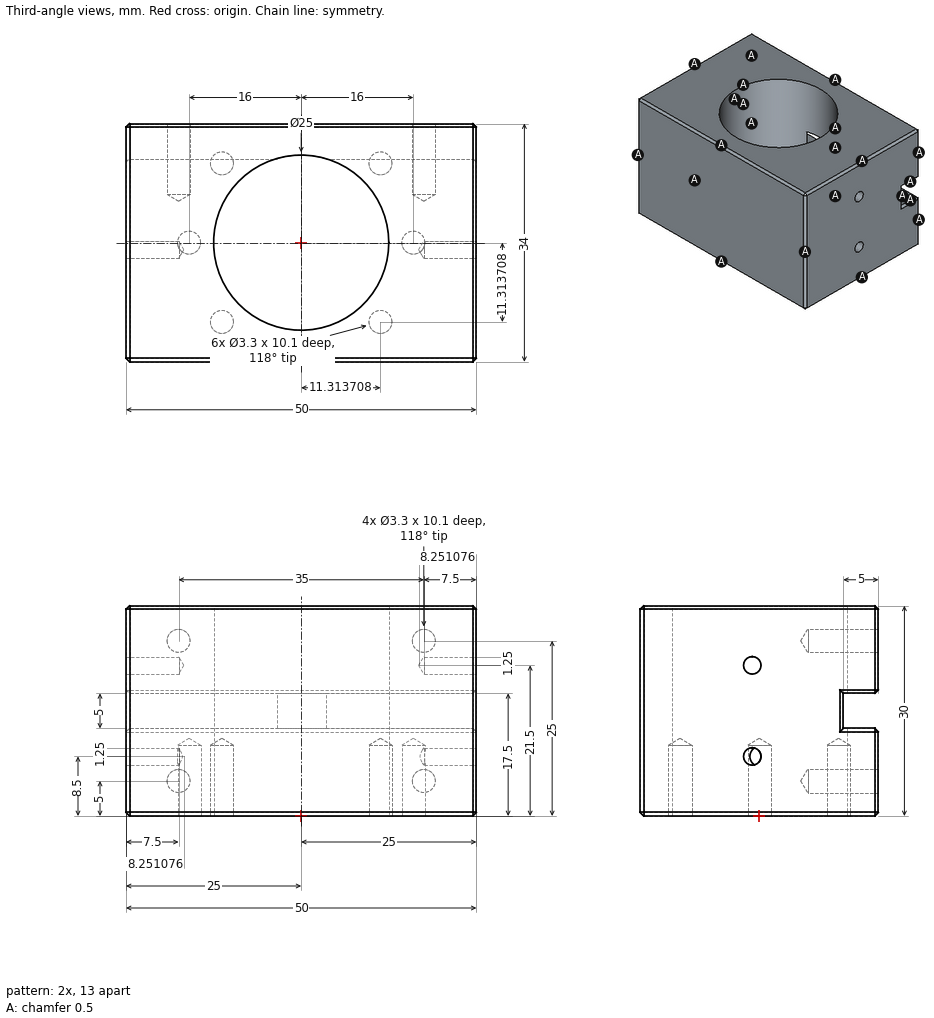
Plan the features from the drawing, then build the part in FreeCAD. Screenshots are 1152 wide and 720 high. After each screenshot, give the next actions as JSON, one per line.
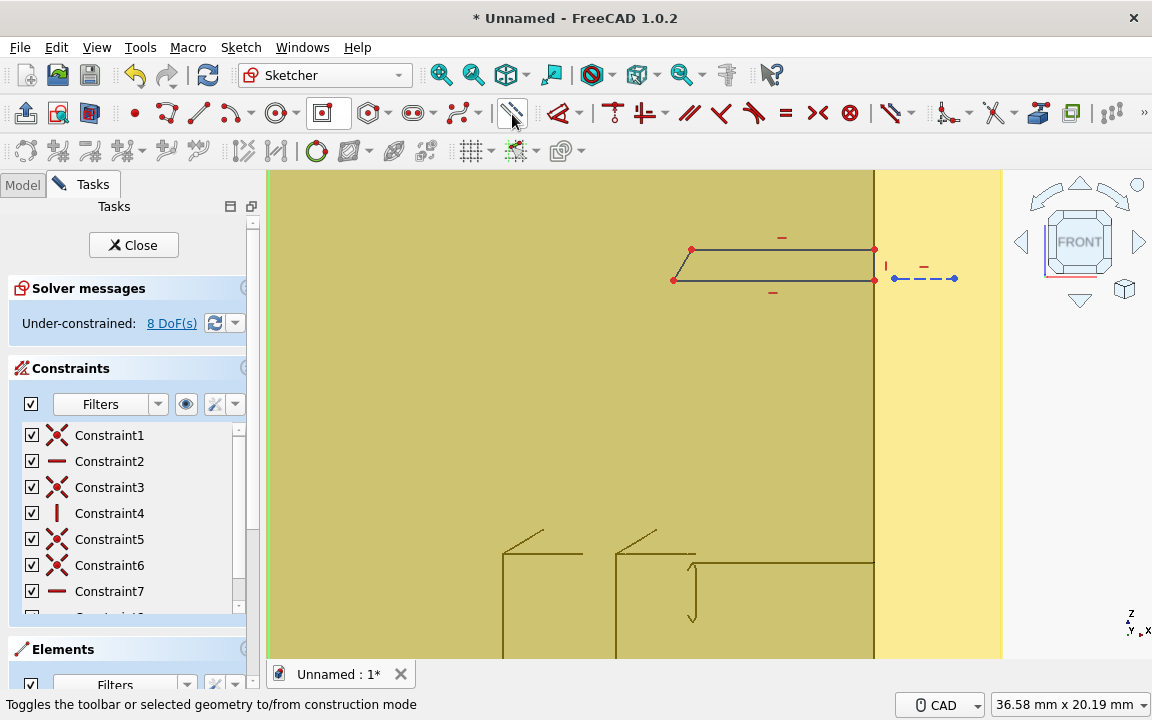
{"action": "left_click", "coordinate": [747, 250]}
{"action": "left_click", "coordinate": [783, 216]}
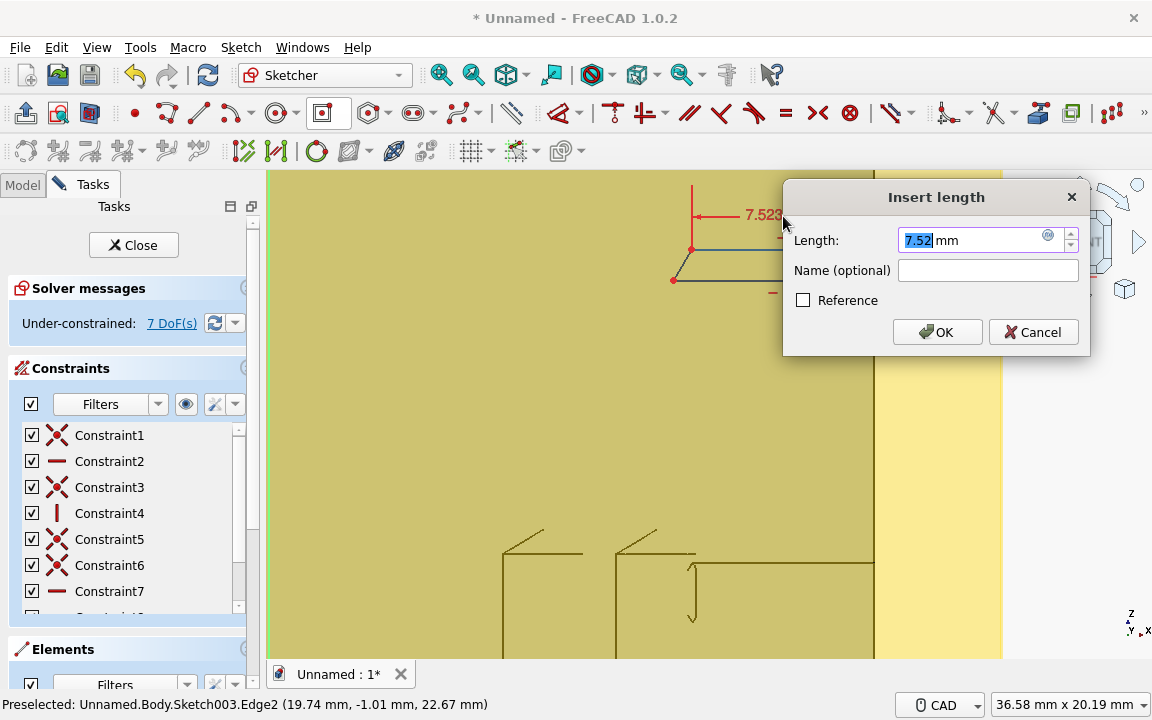
{"action": "type", "text": "7.5"}
{"action": "key", "text": "Return"}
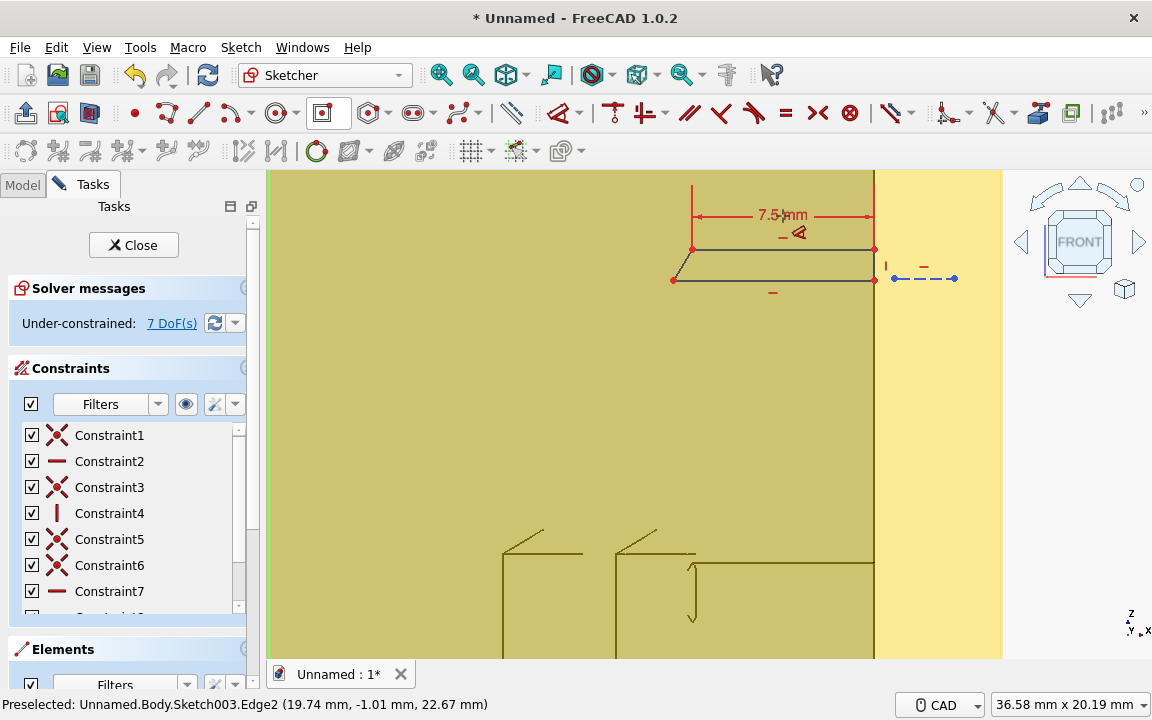
{"action": "left_click", "coordinate": [874, 250]}
{"action": "left_click", "coordinate": [584, 216]}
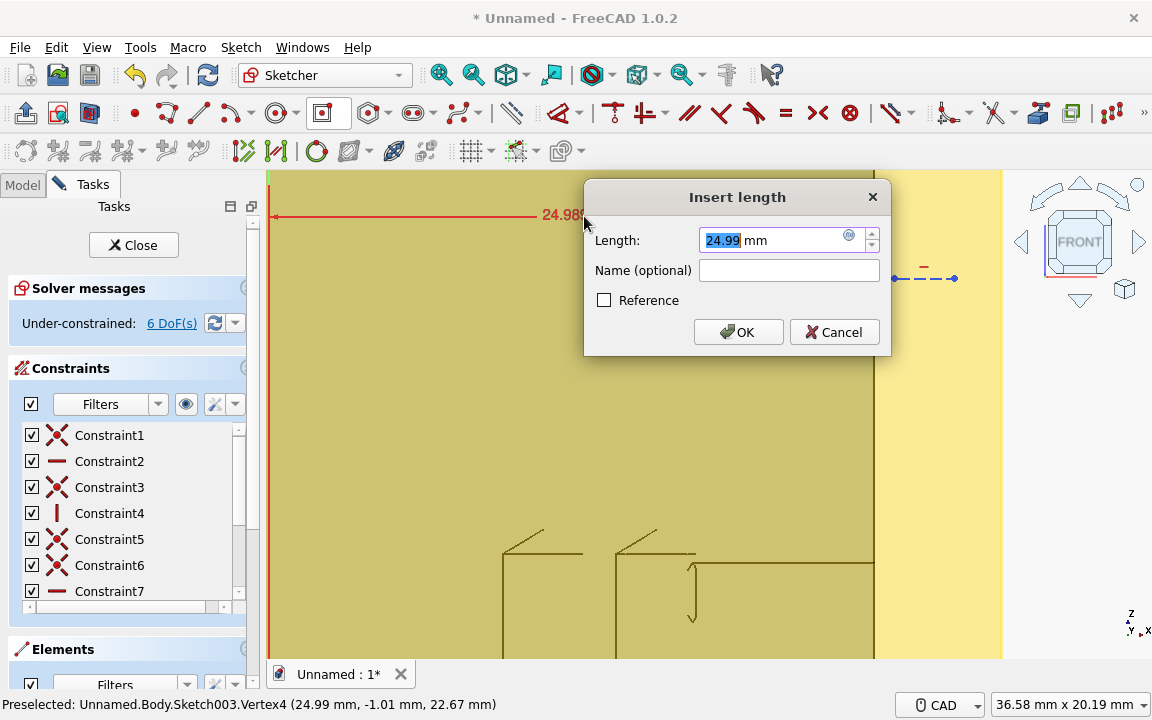
{"action": "type", "text": "25"}
{"action": "key", "text": "Return"}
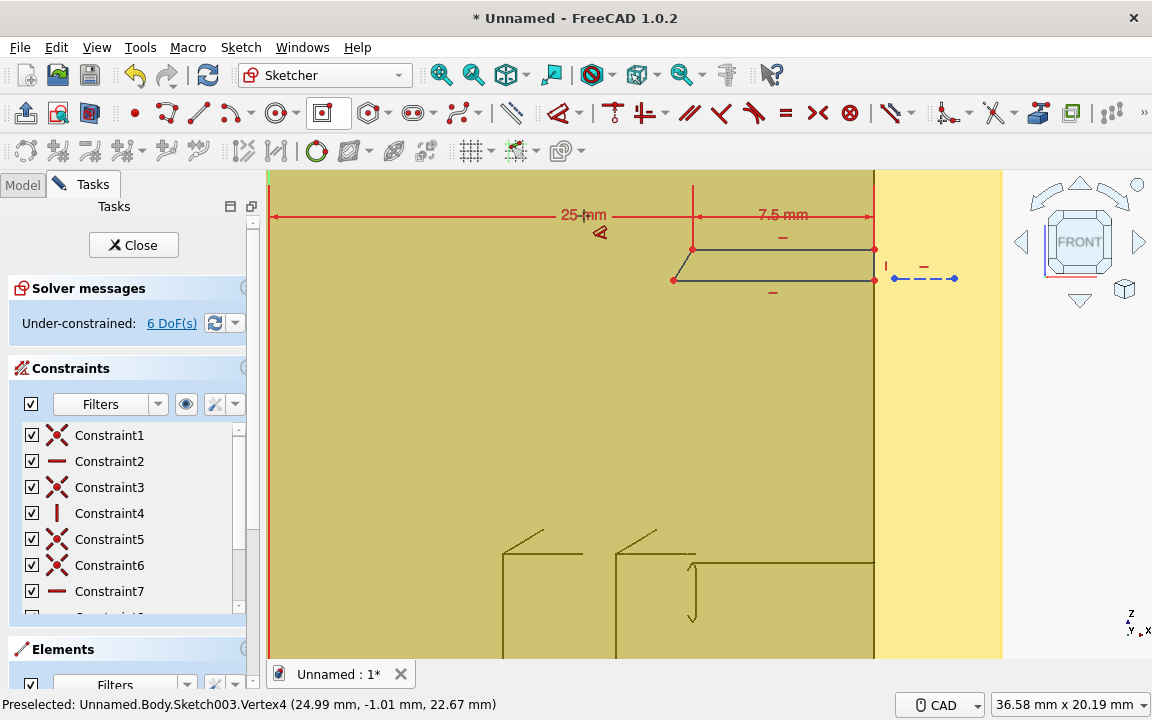
{"action": "scroll", "coordinate": [874, 259], "scroll_direction": "up", "scroll_amount": 2}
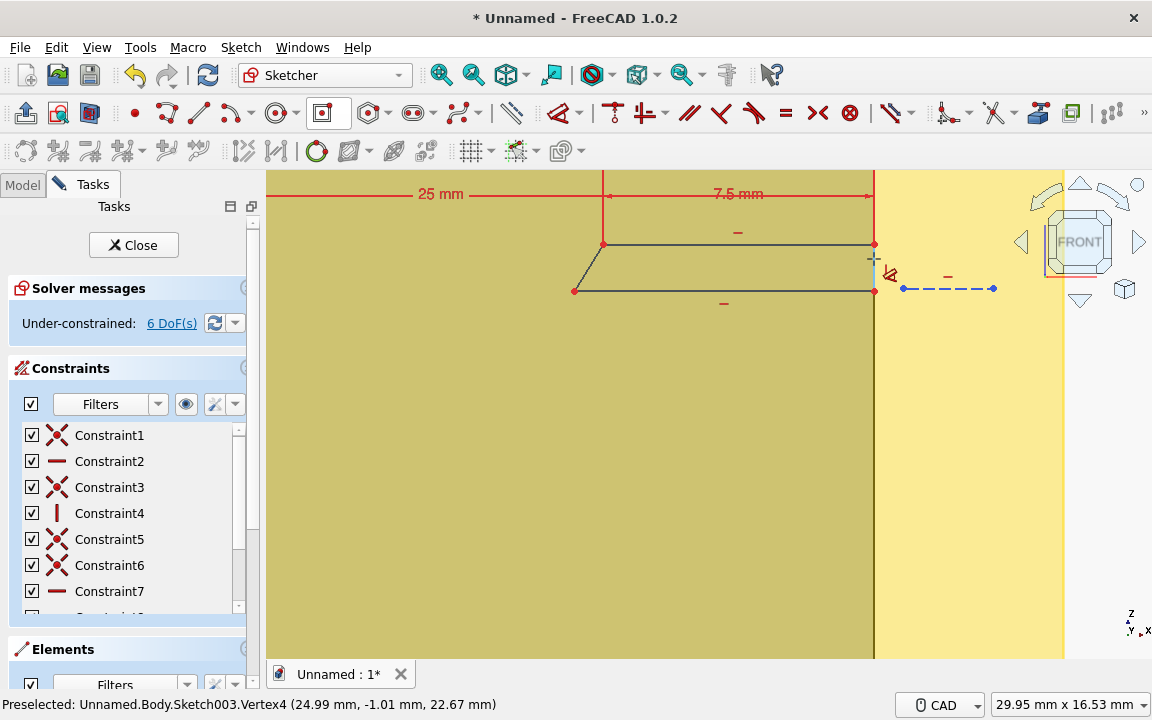
{"action": "left_click", "coordinate": [874, 259]}
{"action": "left_click", "coordinate": [908, 268]}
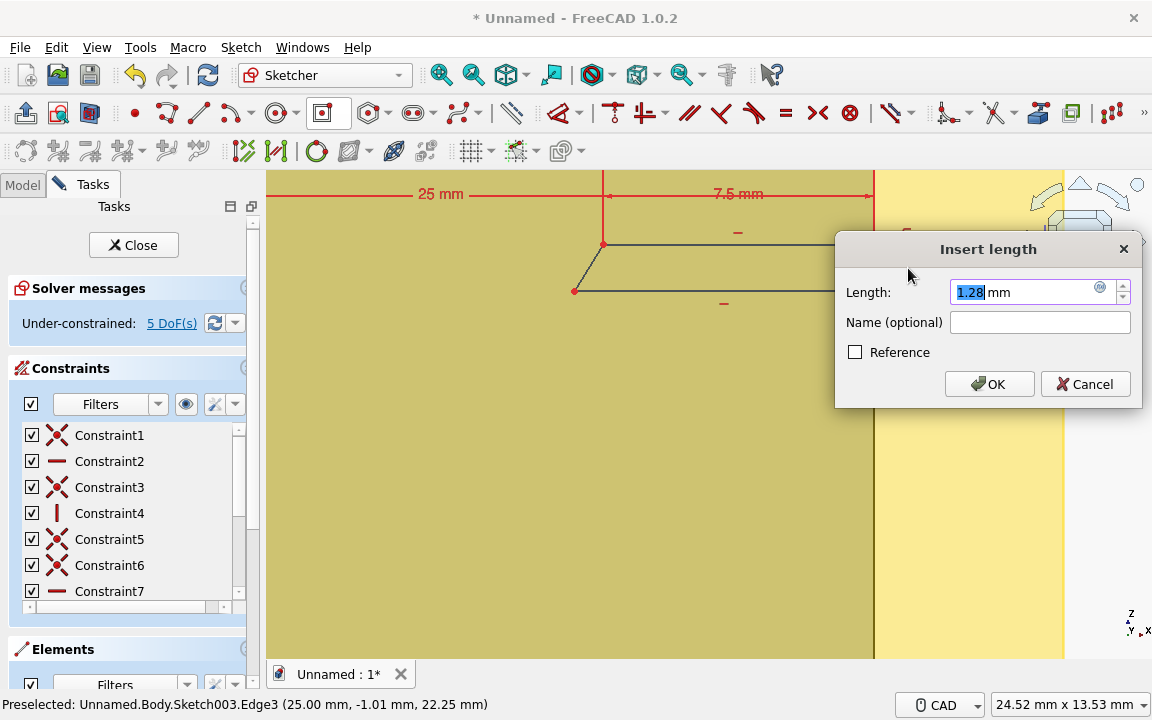
{"action": "type", "text": "1.25"}
{"action": "key", "text": "Return"}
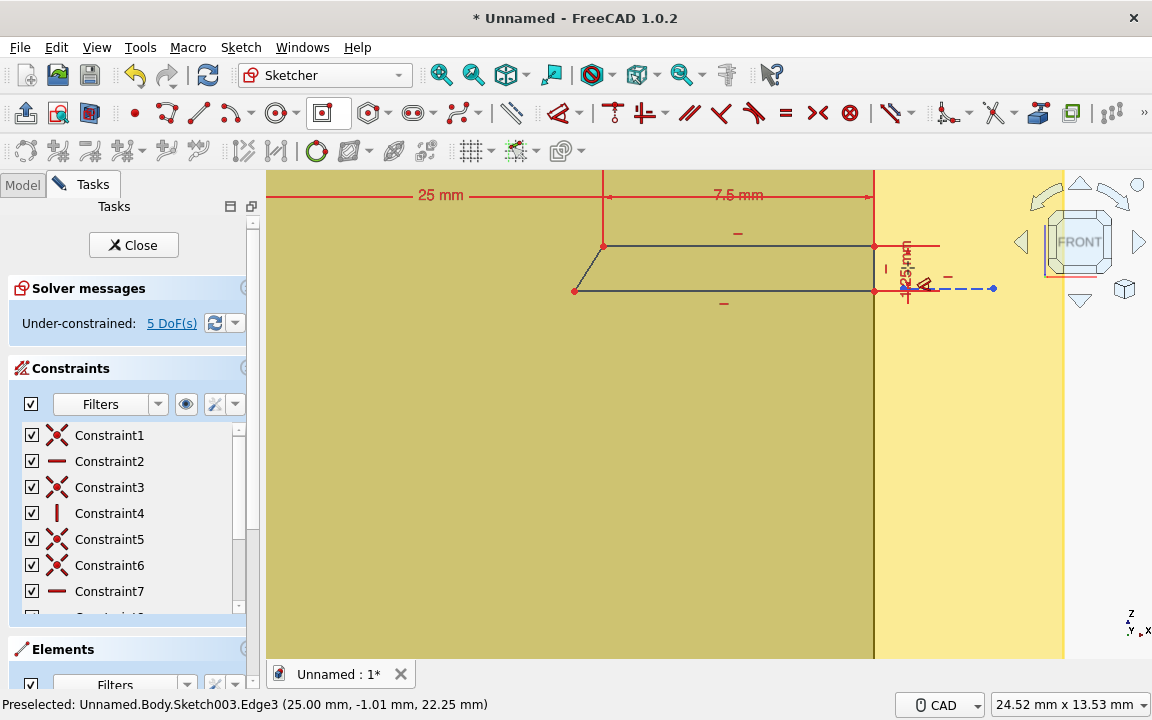
{"action": "left_click", "coordinate": [575, 291]}
{"action": "left_click", "coordinate": [609, 461]}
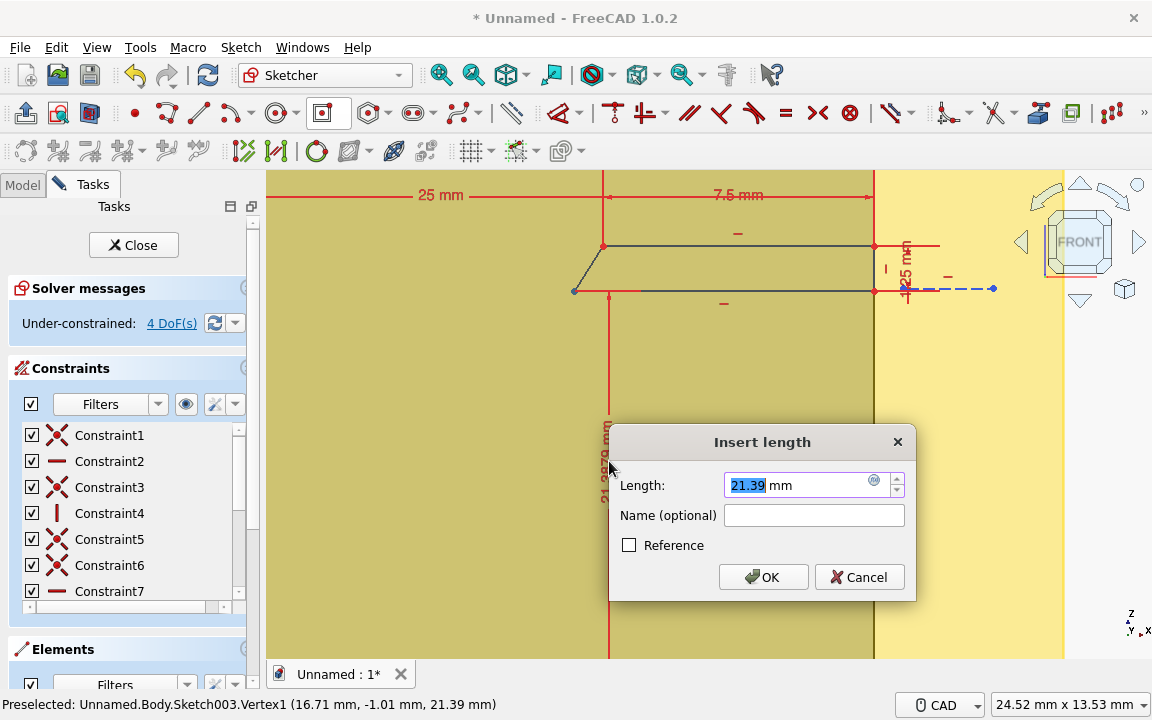
{"action": "type", "text": "21.5"}
{"action": "key", "text": "Return"}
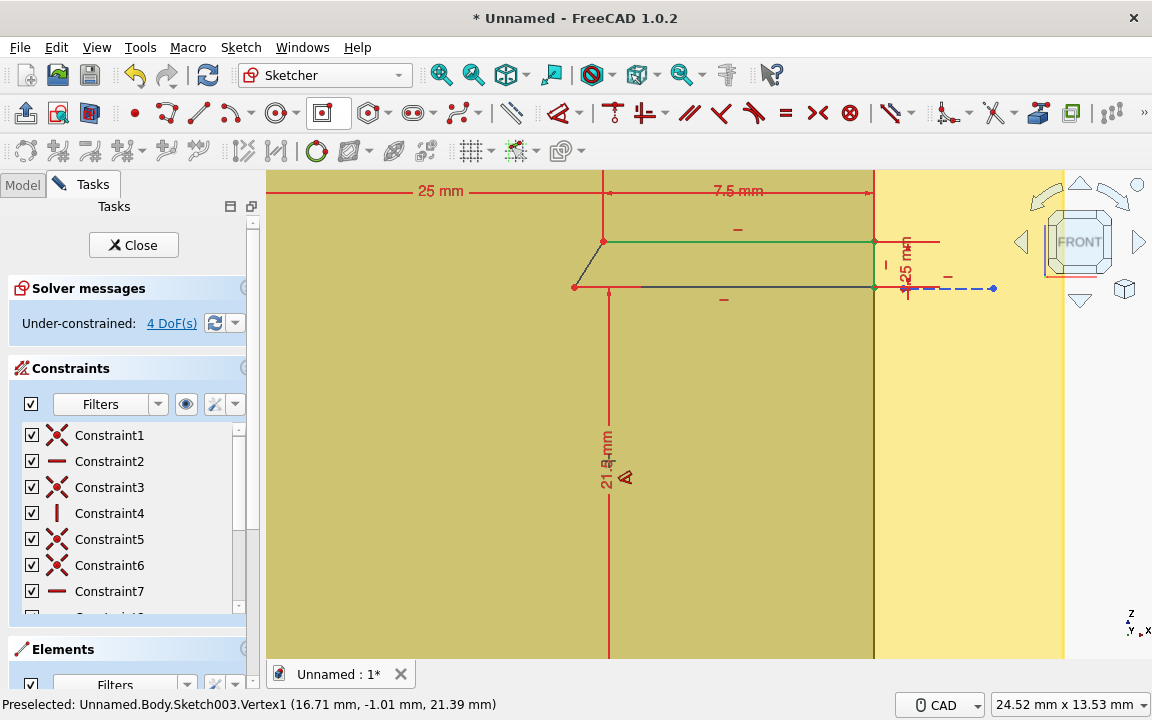
{"action": "left_click", "coordinate": [903, 289]}
{"action": "left_click", "coordinate": [937, 460]}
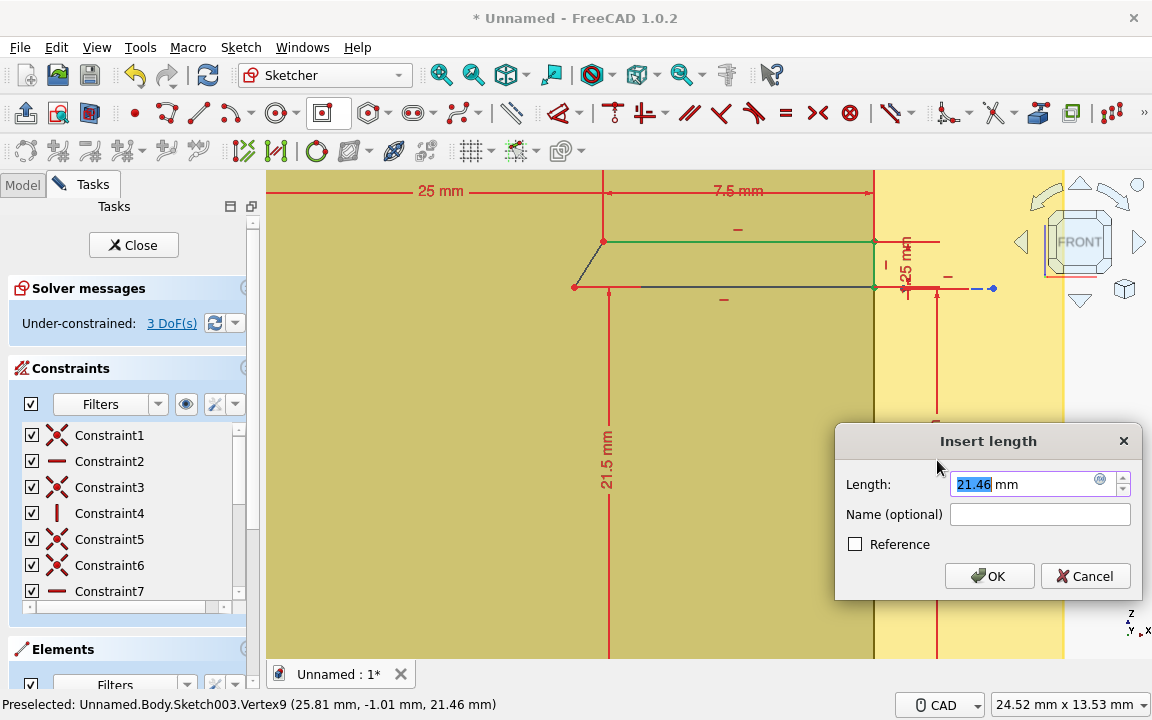
{"action": "type", "text": "21.5"}
{"action": "key", "text": "Return"}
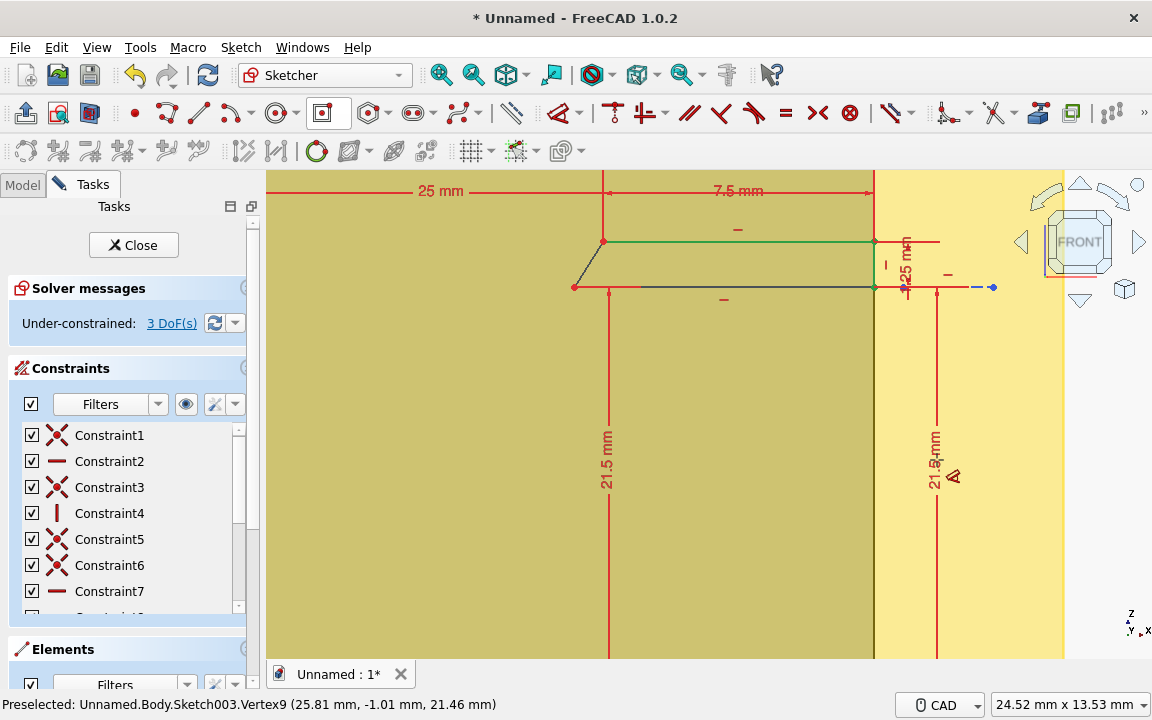
{"action": "left_click", "coordinate": [784, 287]}
{"action": "left_click", "coordinate": [724, 321]}